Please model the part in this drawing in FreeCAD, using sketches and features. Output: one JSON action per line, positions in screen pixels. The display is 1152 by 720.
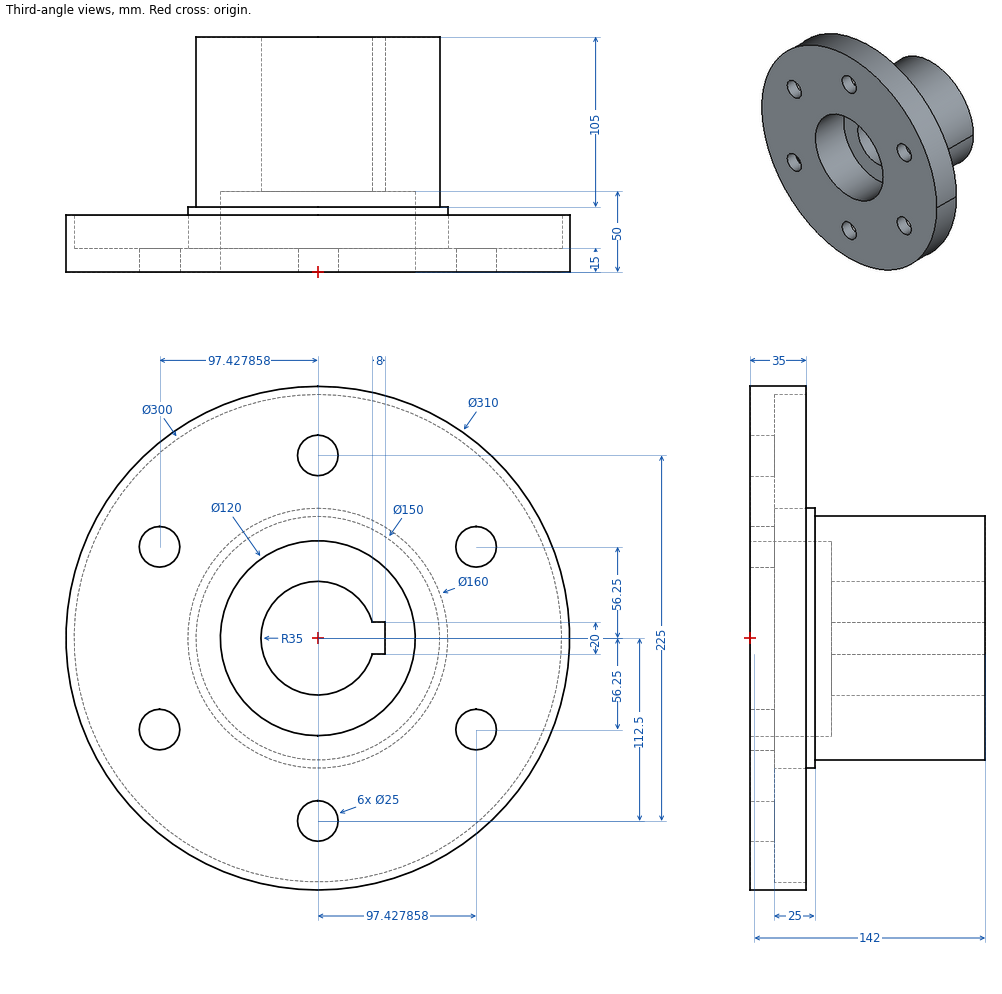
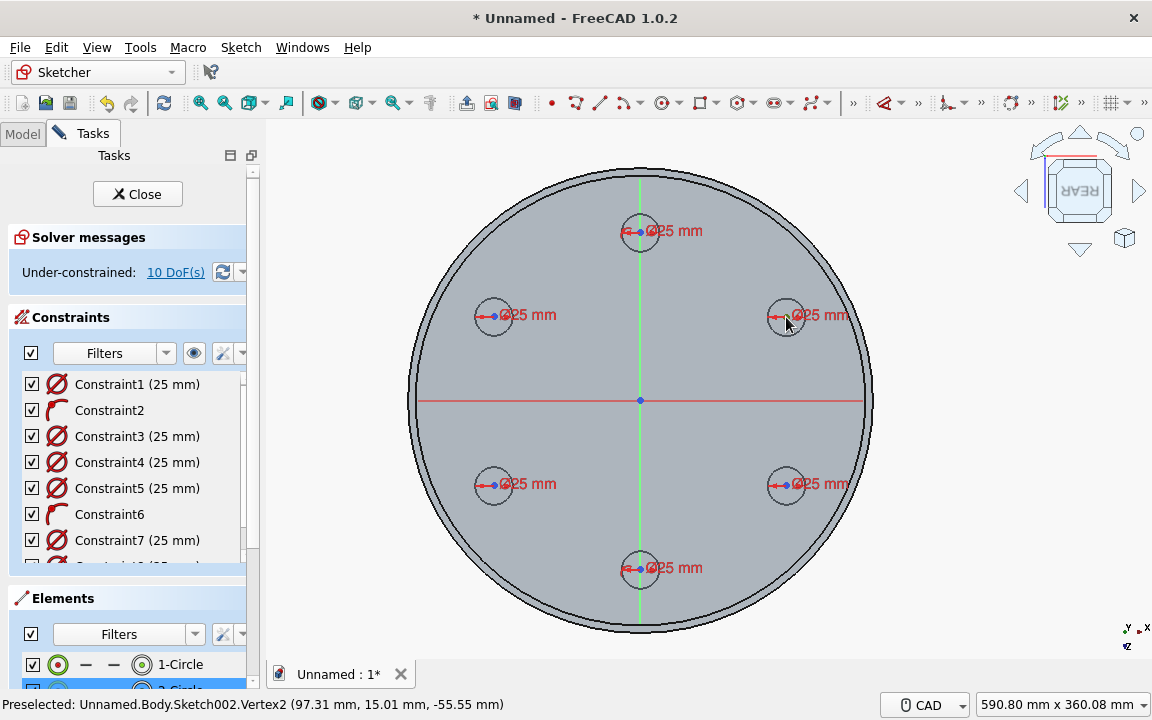
{"action": "left_click", "coordinate": [786, 486]}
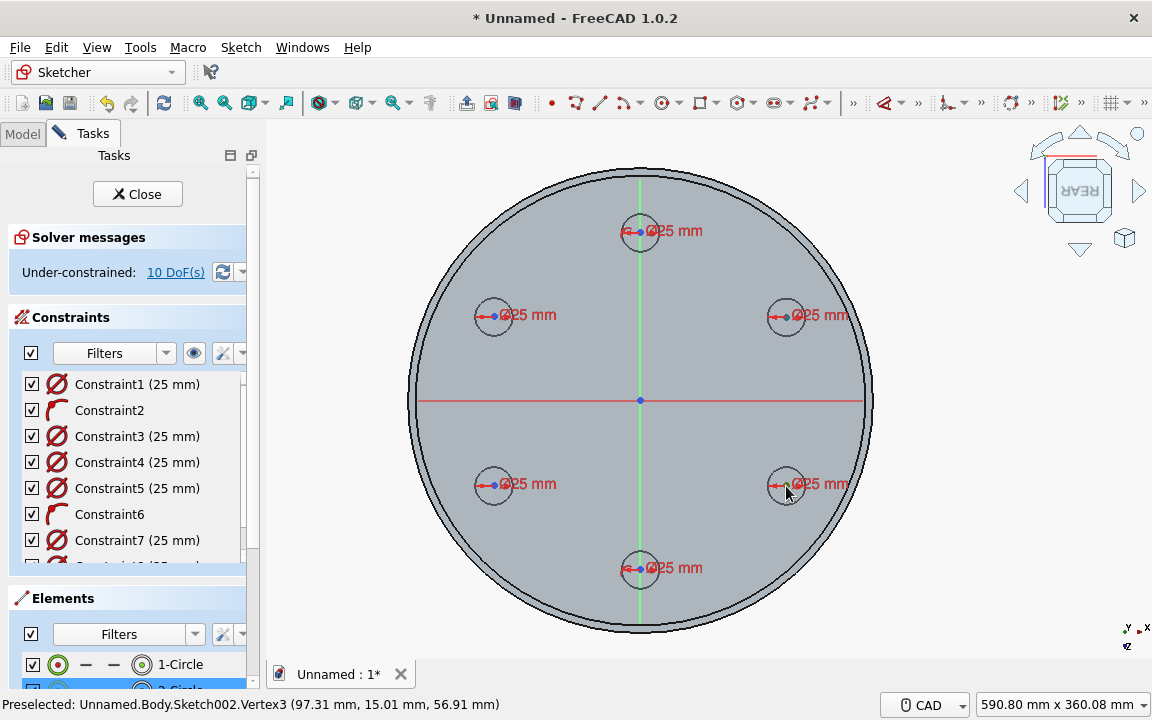
{"action": "key", "text": "v"}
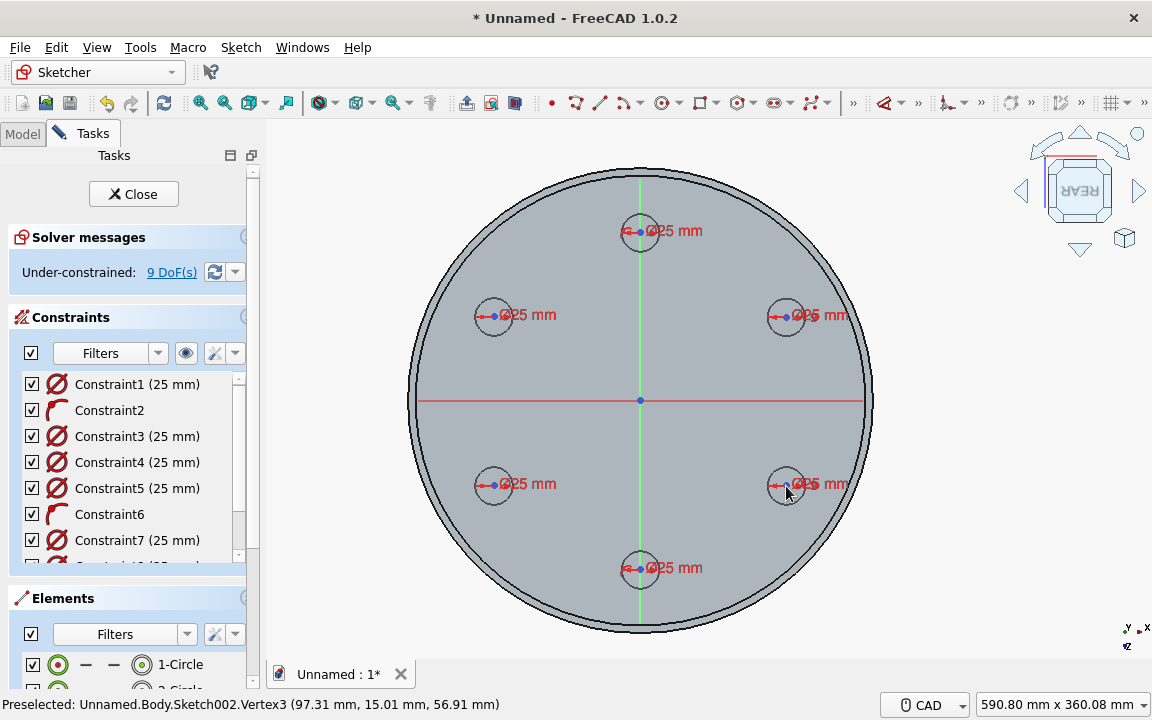
{"action": "left_click", "coordinate": [786, 486]}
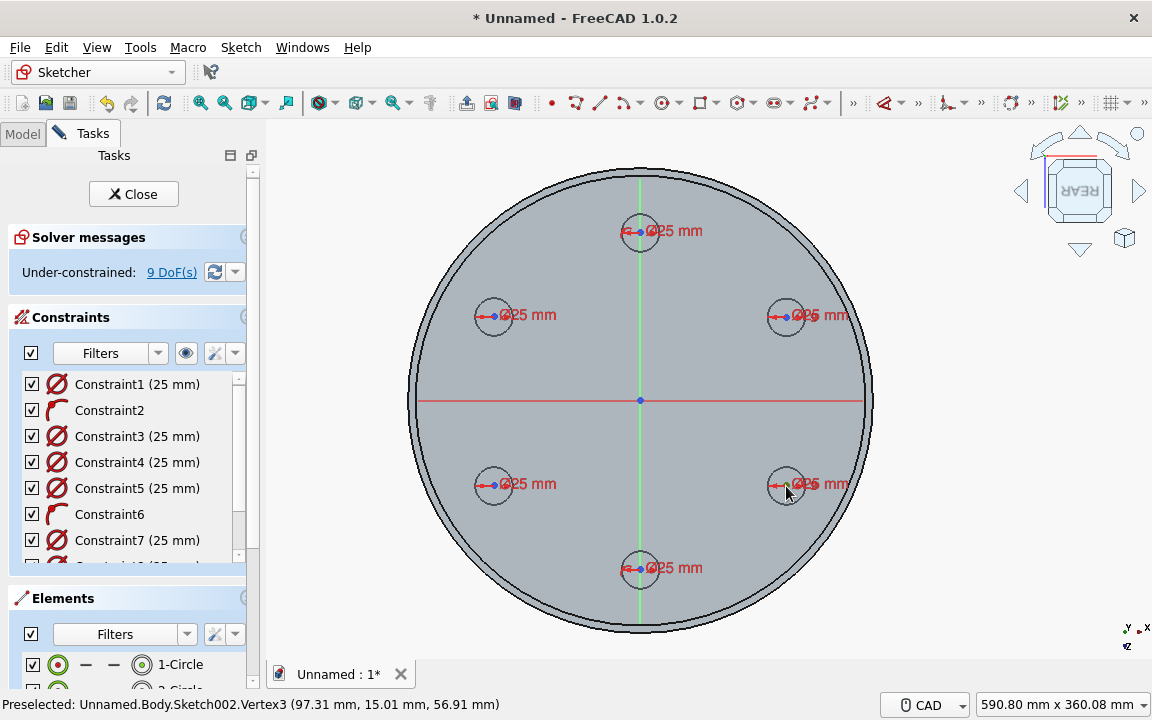
{"action": "left_click", "coordinate": [494, 486]}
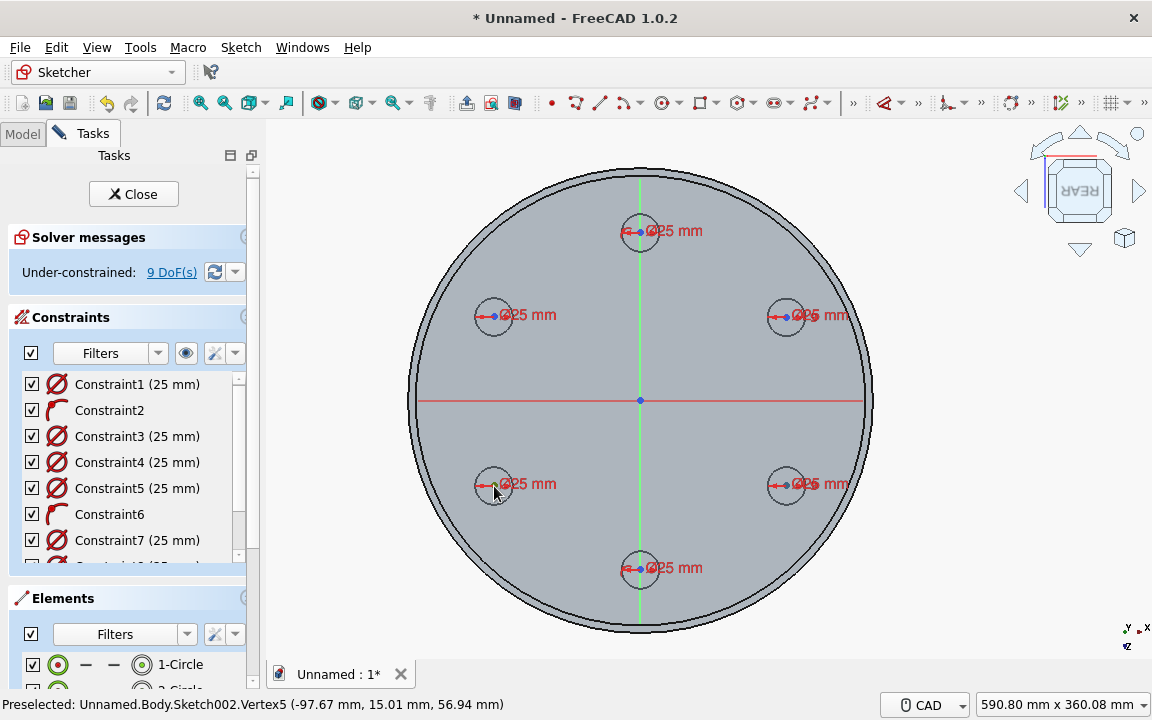
{"action": "key", "text": "h"}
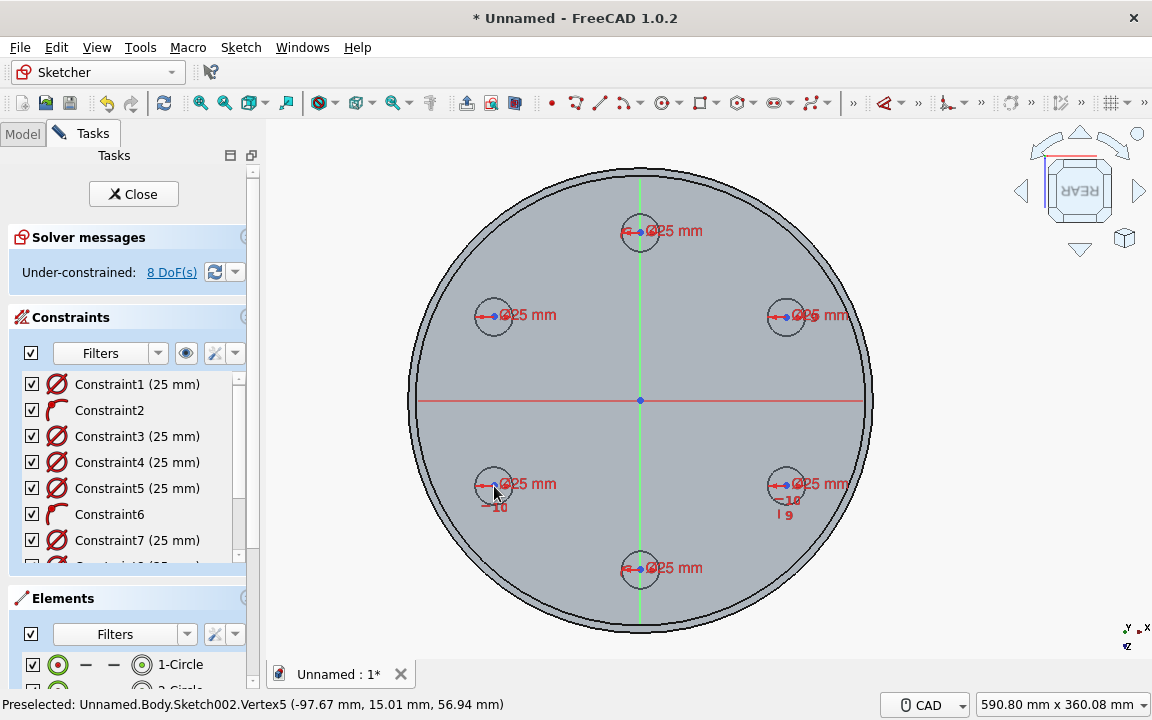
{"action": "left_click", "coordinate": [494, 486]}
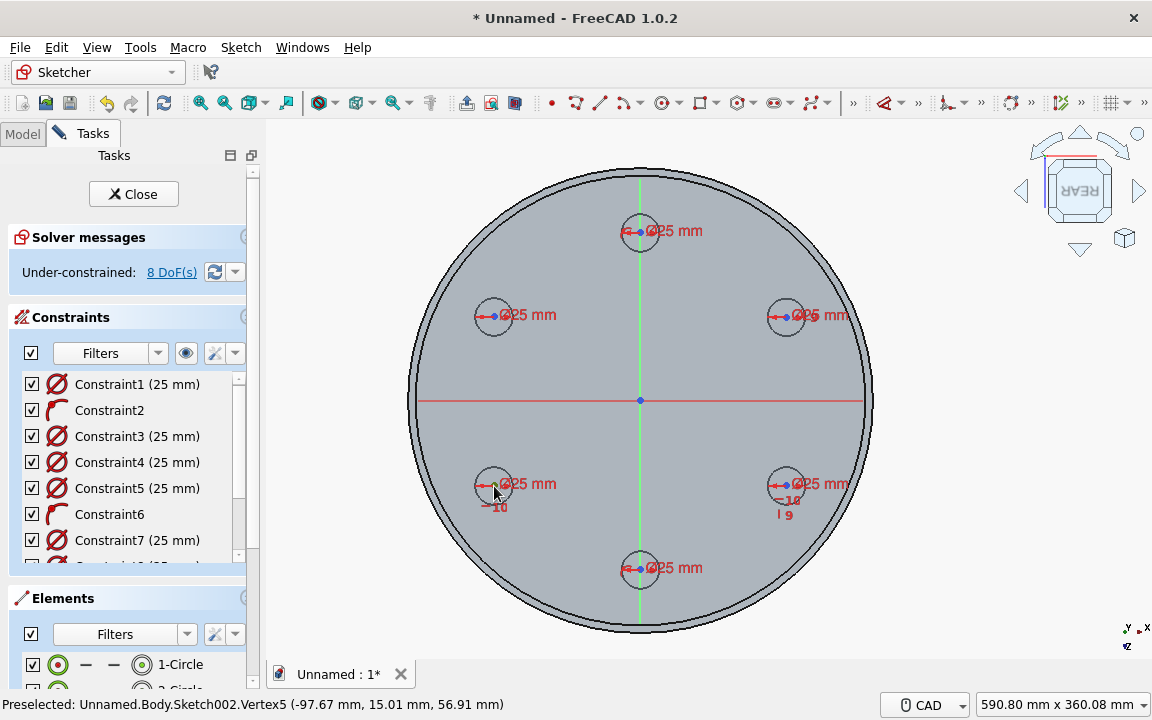
{"action": "left_click", "coordinate": [494, 317]}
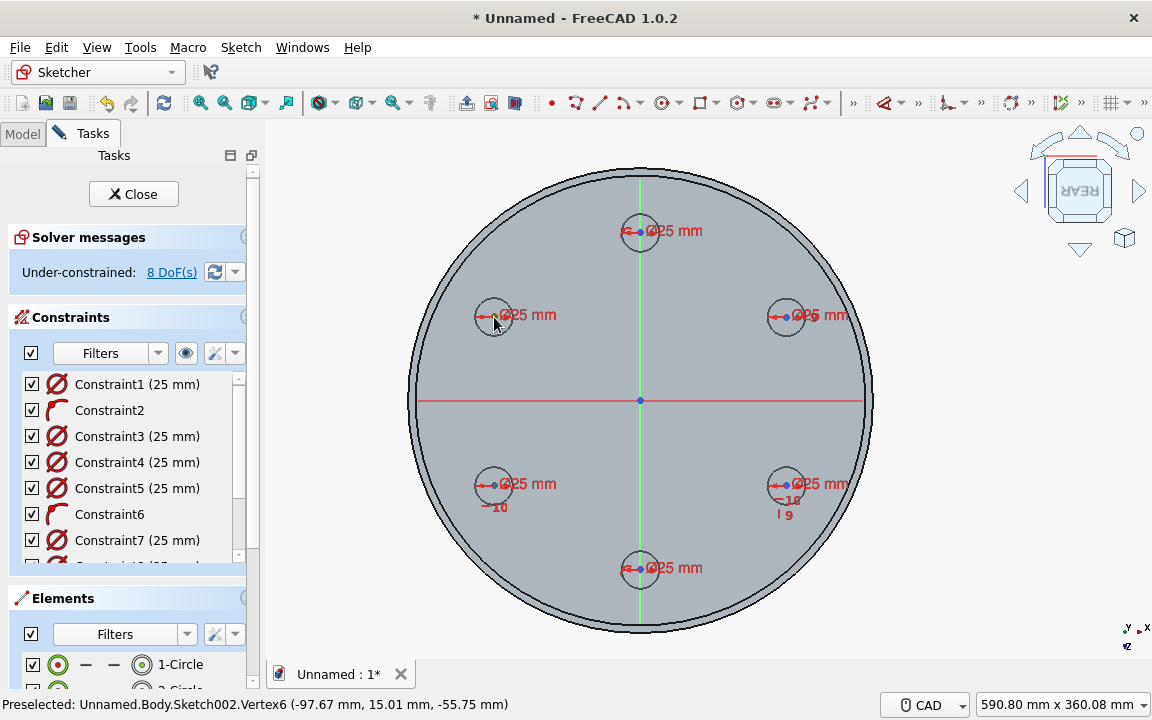
{"action": "key", "text": "v"}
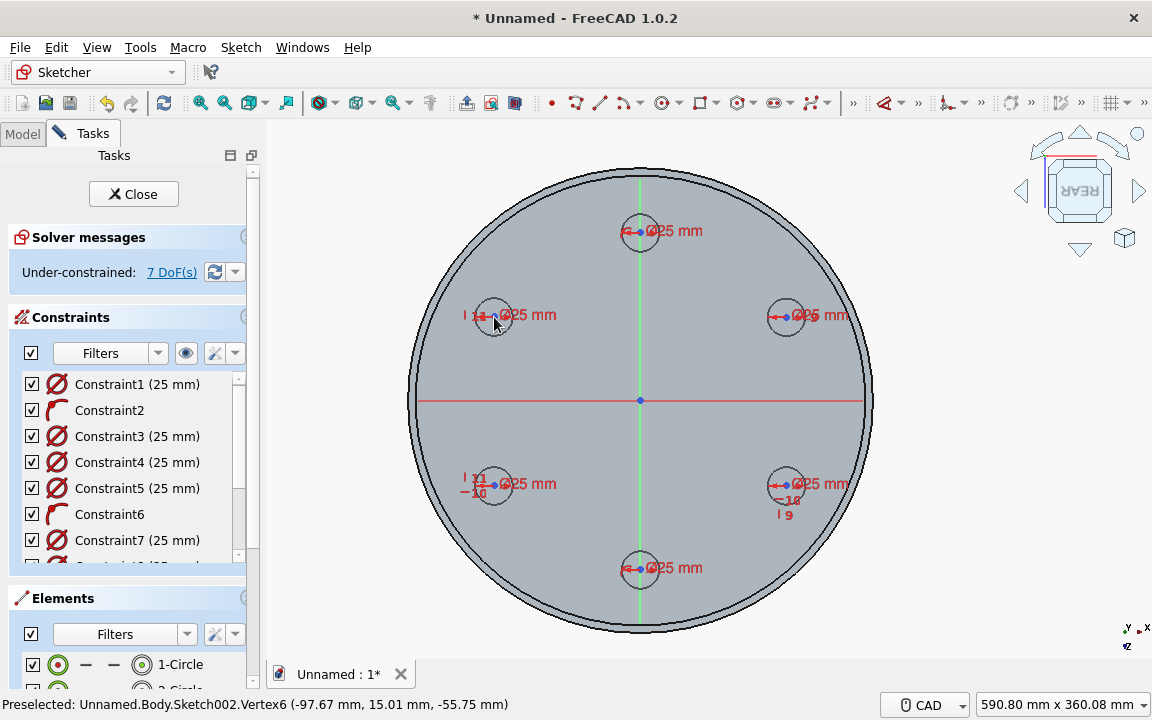
{"action": "left_click", "coordinate": [786, 317]}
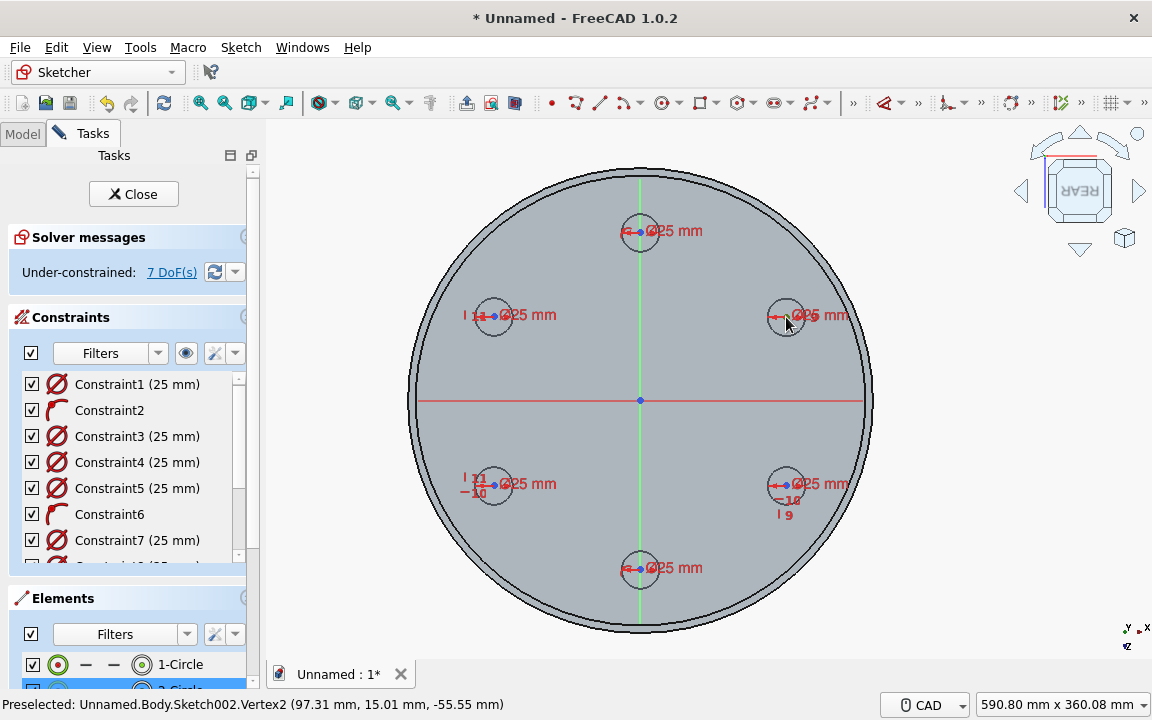
{"action": "left_click", "coordinate": [494, 317]}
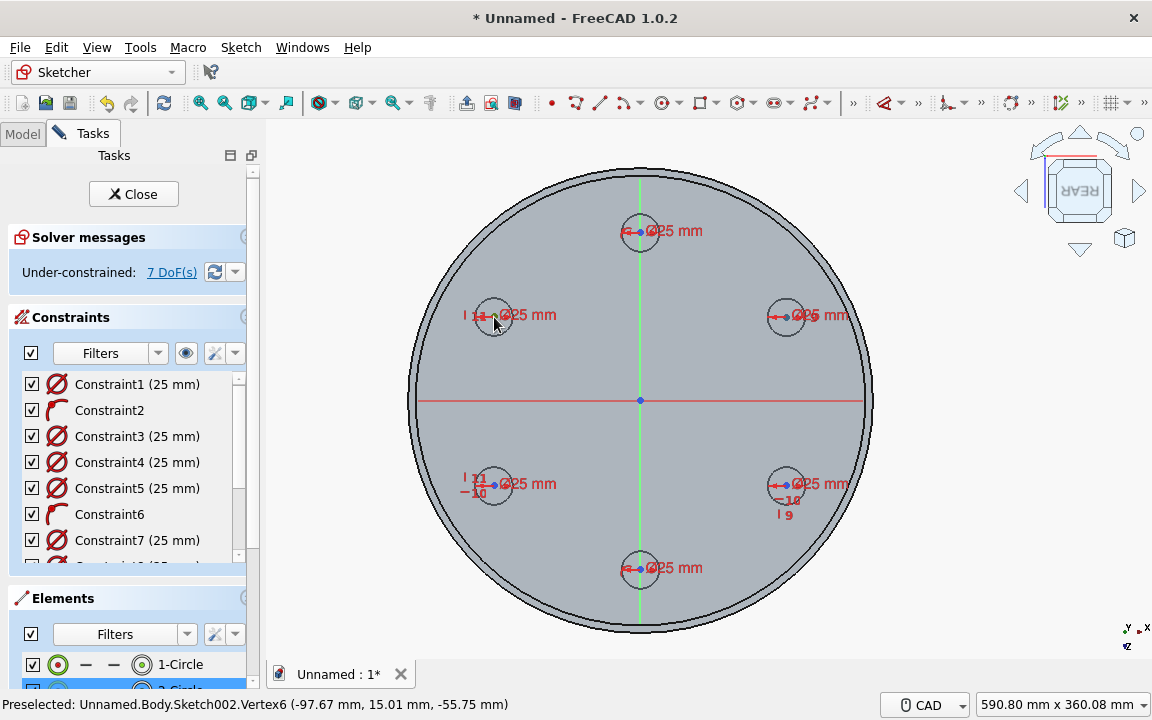
{"action": "key", "text": "h"}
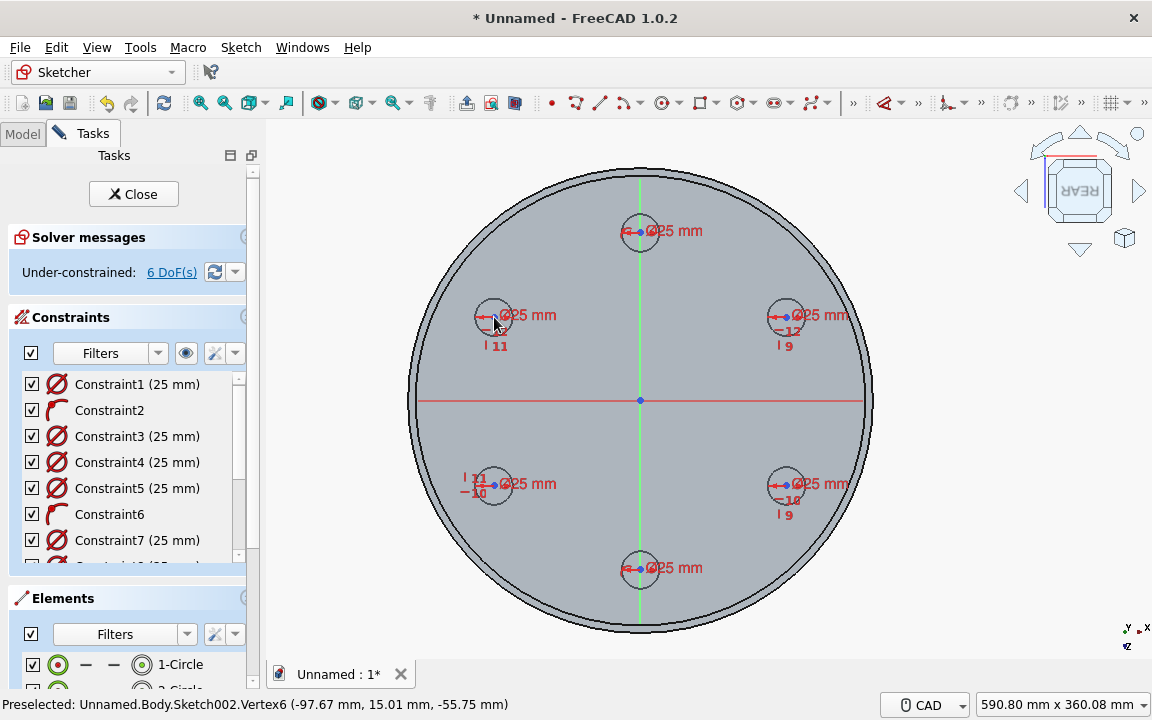
{"action": "left_click", "coordinate": [884, 104]}